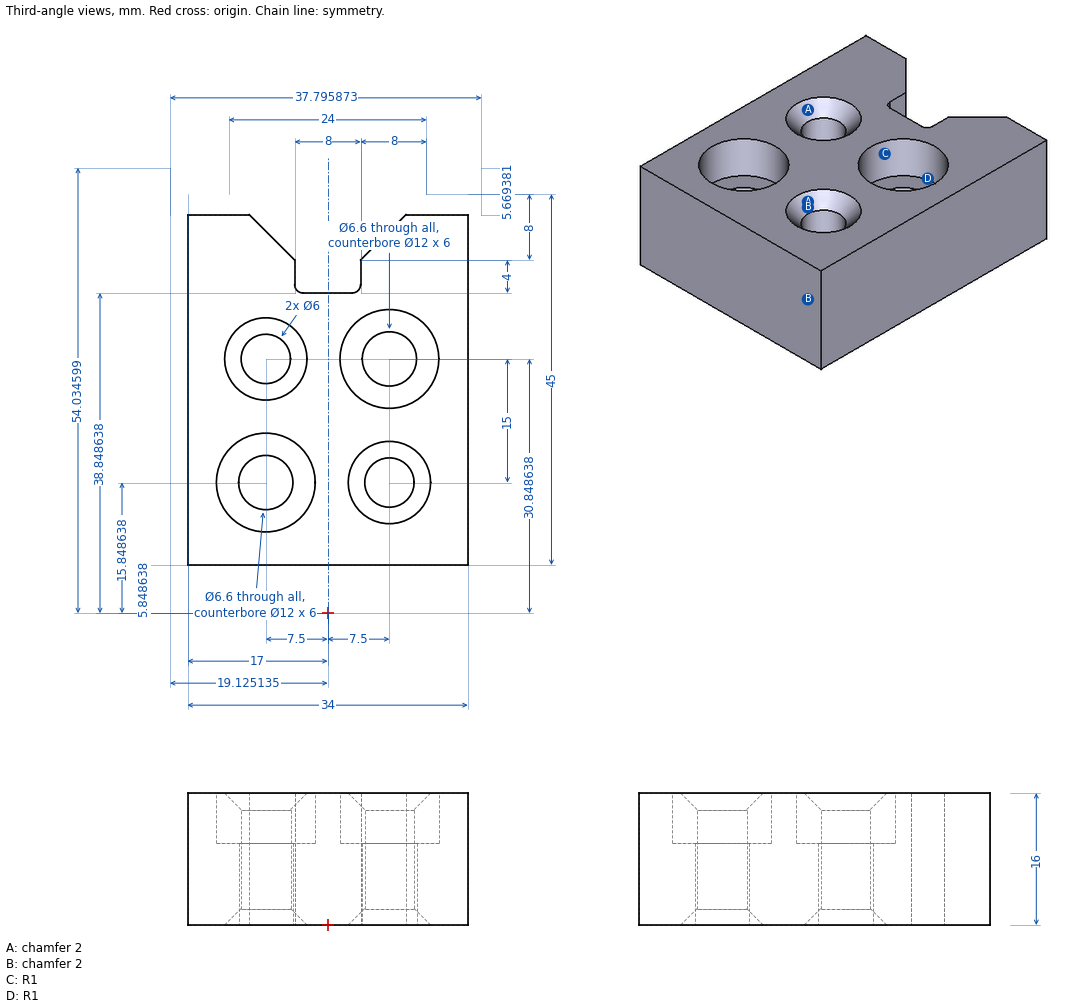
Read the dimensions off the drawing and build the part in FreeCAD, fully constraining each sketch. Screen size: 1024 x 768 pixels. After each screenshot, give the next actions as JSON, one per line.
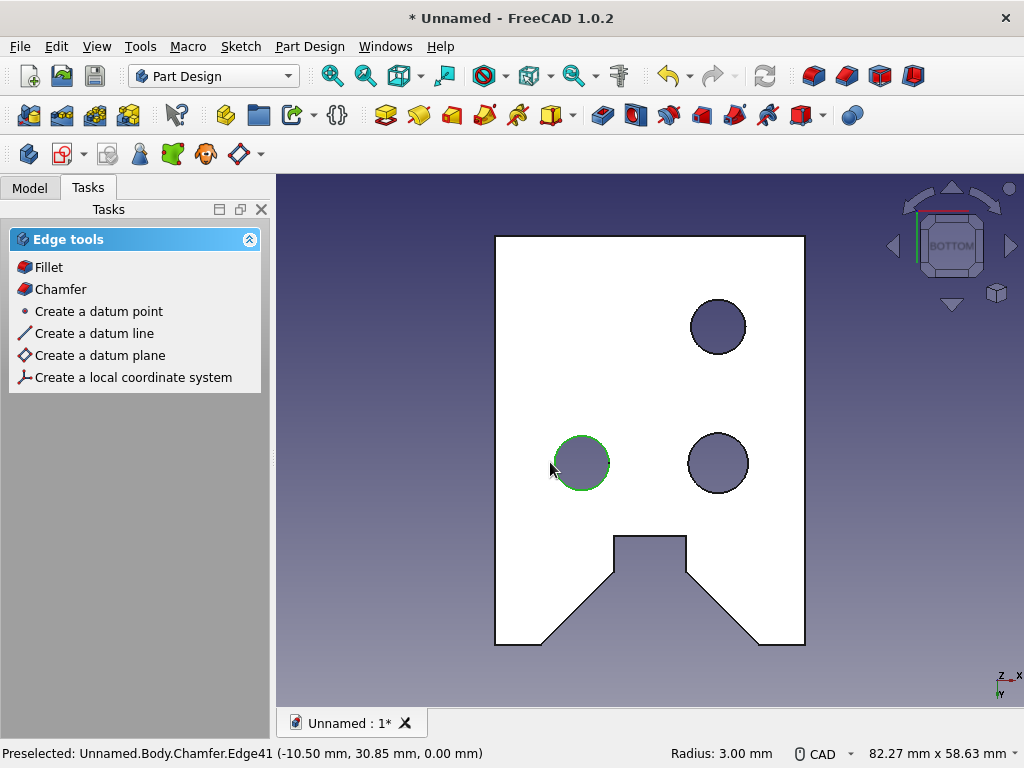
{"action": "left_click", "coordinate": [691, 326], "text": "ctrl"}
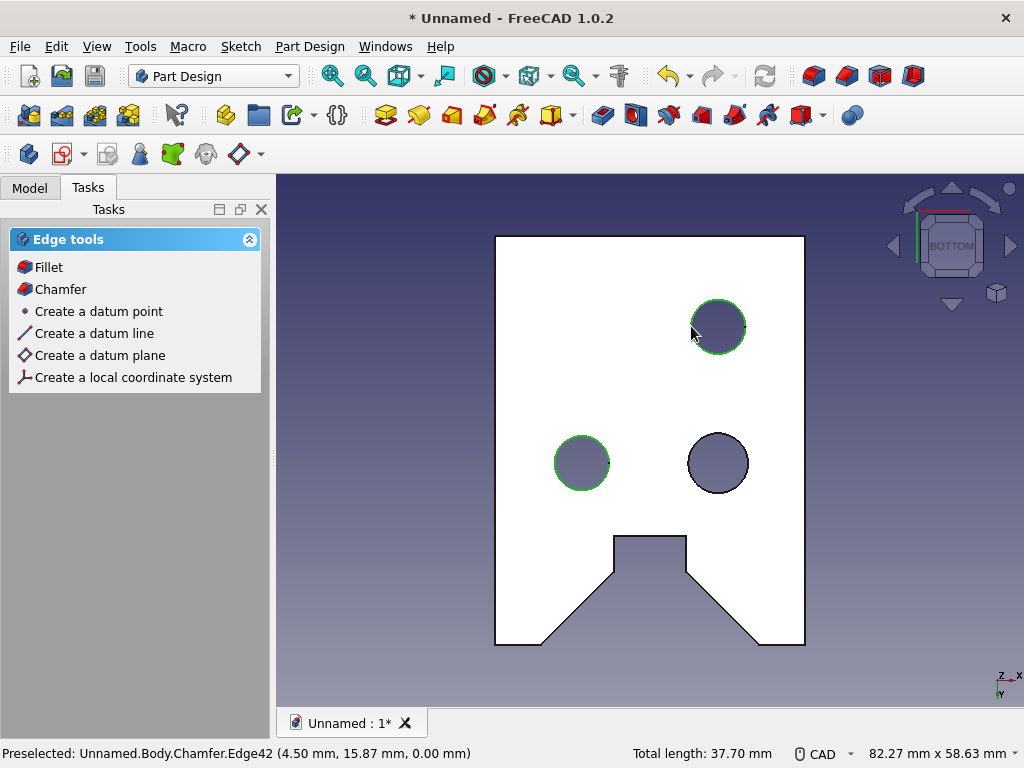
{"action": "left_click", "coordinate": [847, 76]}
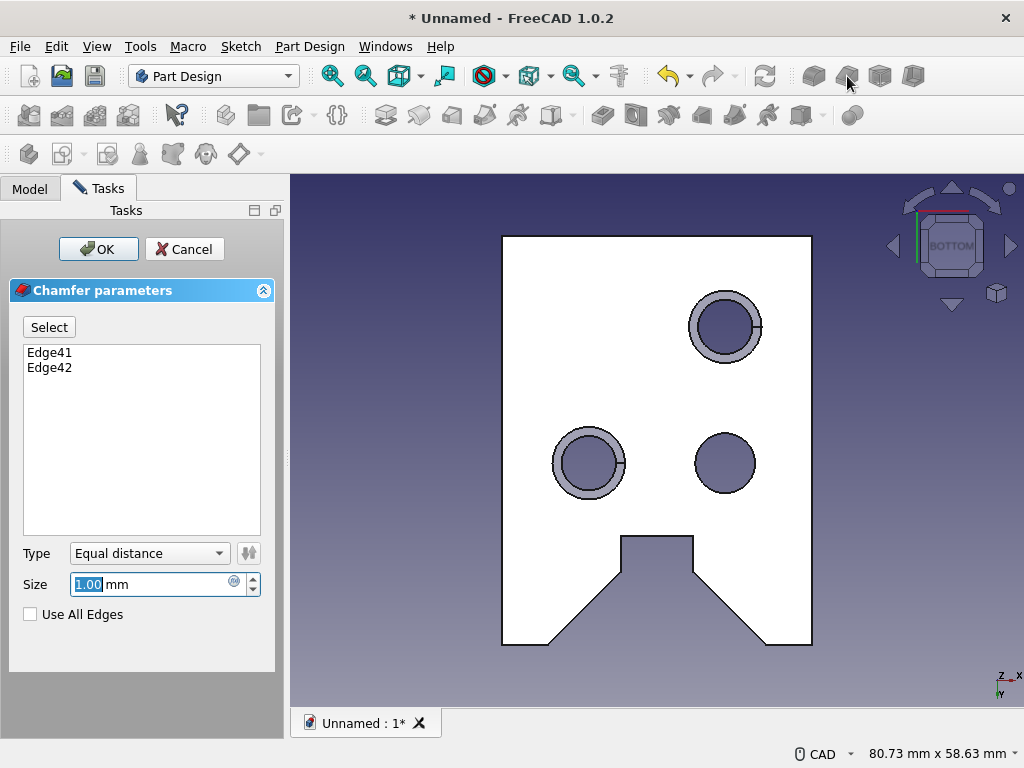
{"action": "type", "text": "2"}
{"action": "key", "text": "Tab"}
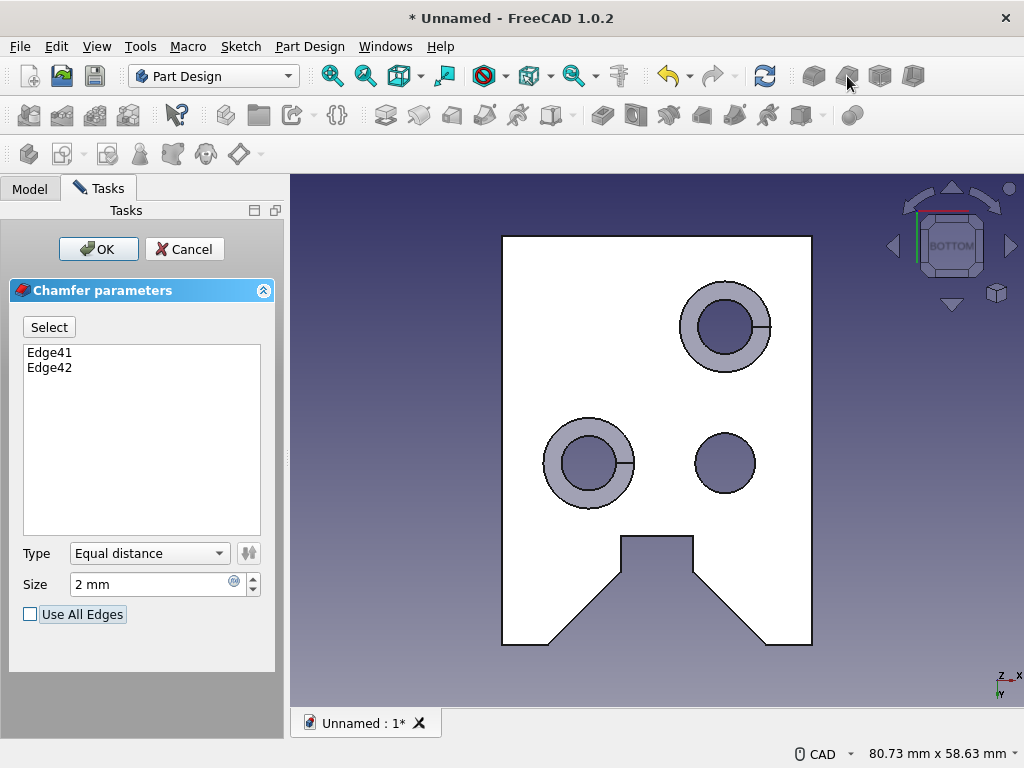
{"action": "left_click", "coordinate": [99, 249]}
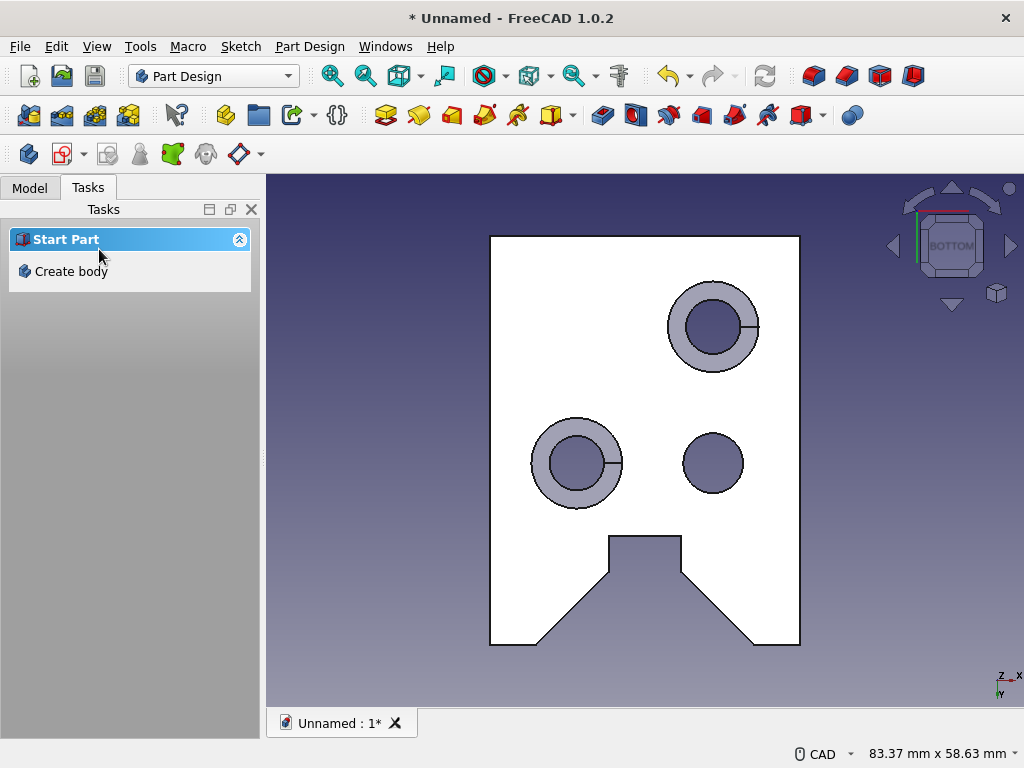
{"action": "key", "text": "0"}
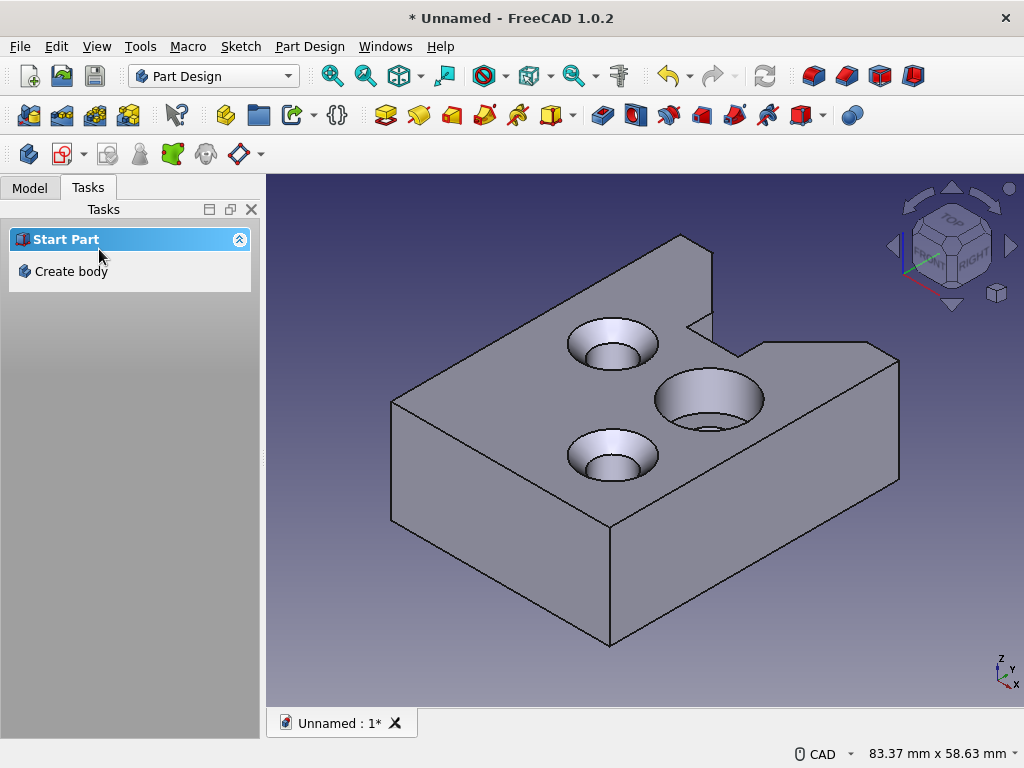
{"action": "left_click", "coordinate": [531, 410]}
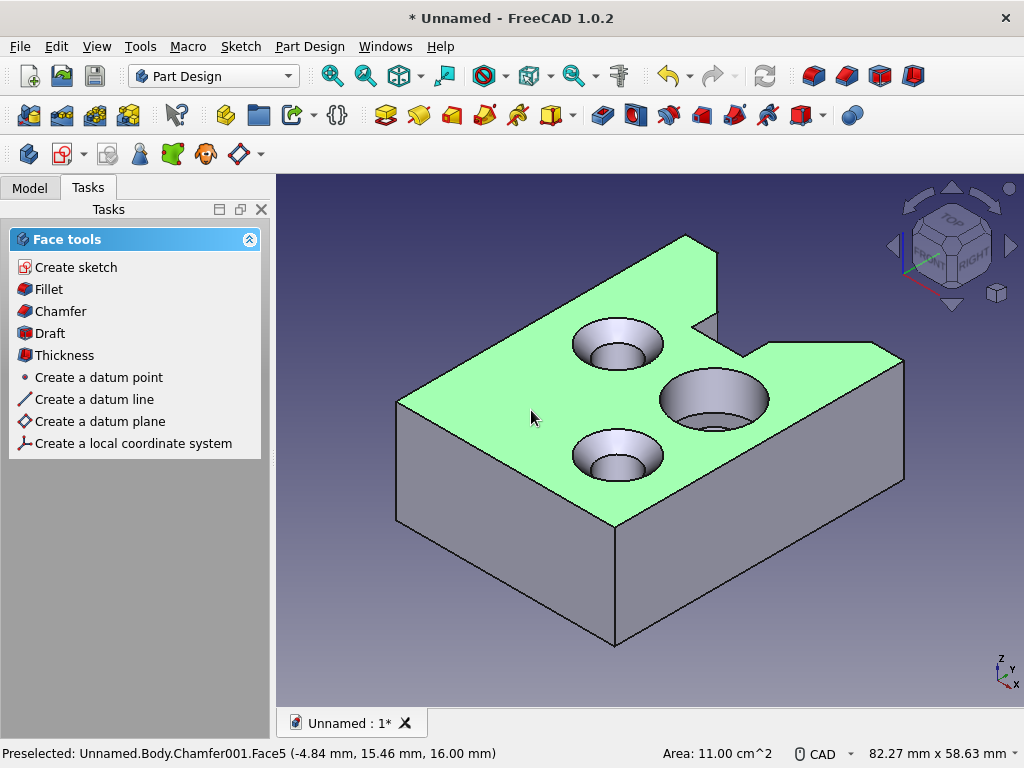
{"action": "left_click", "coordinate": [62, 154]}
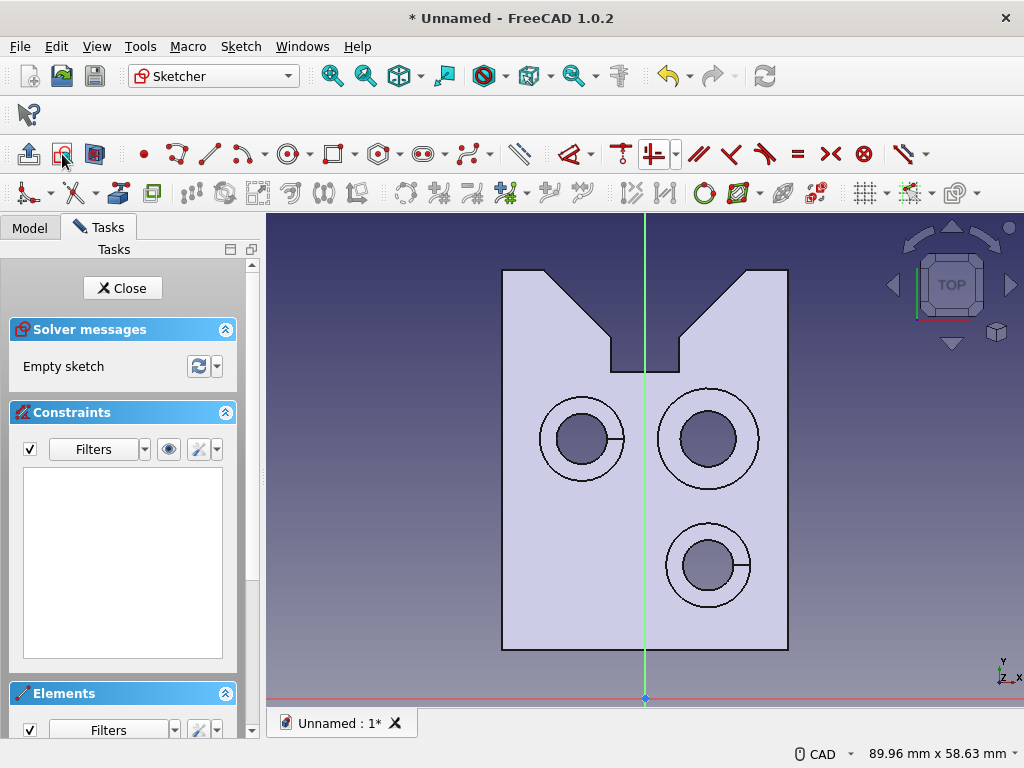
{"action": "scroll", "coordinate": [583, 586], "scroll_direction": "up", "scroll_amount": 9}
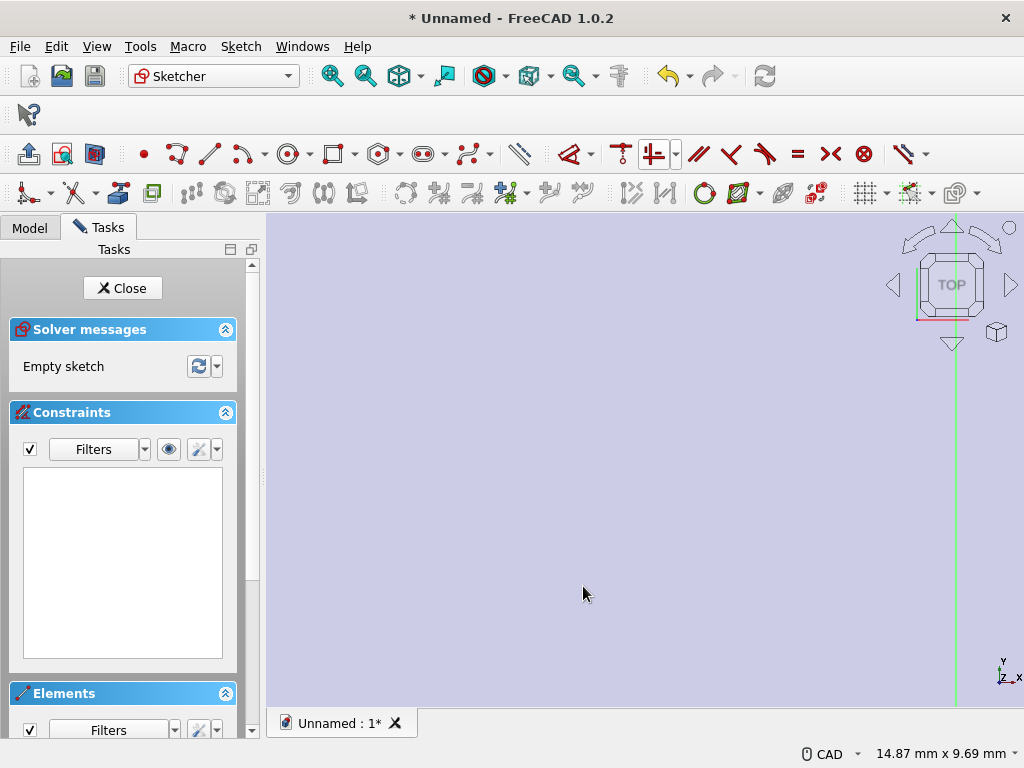
{"action": "left_click", "coordinate": [288, 154]}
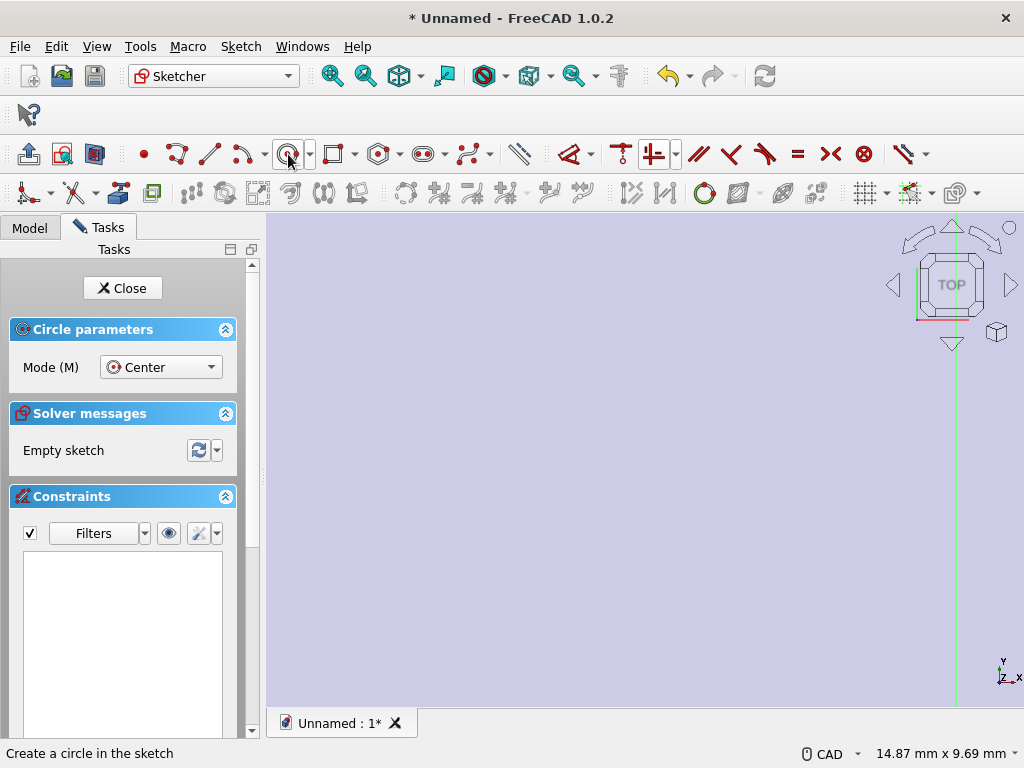
{"action": "left_click", "coordinate": [574, 457]}
{"action": "mouse_move", "coordinate": [693, 338]}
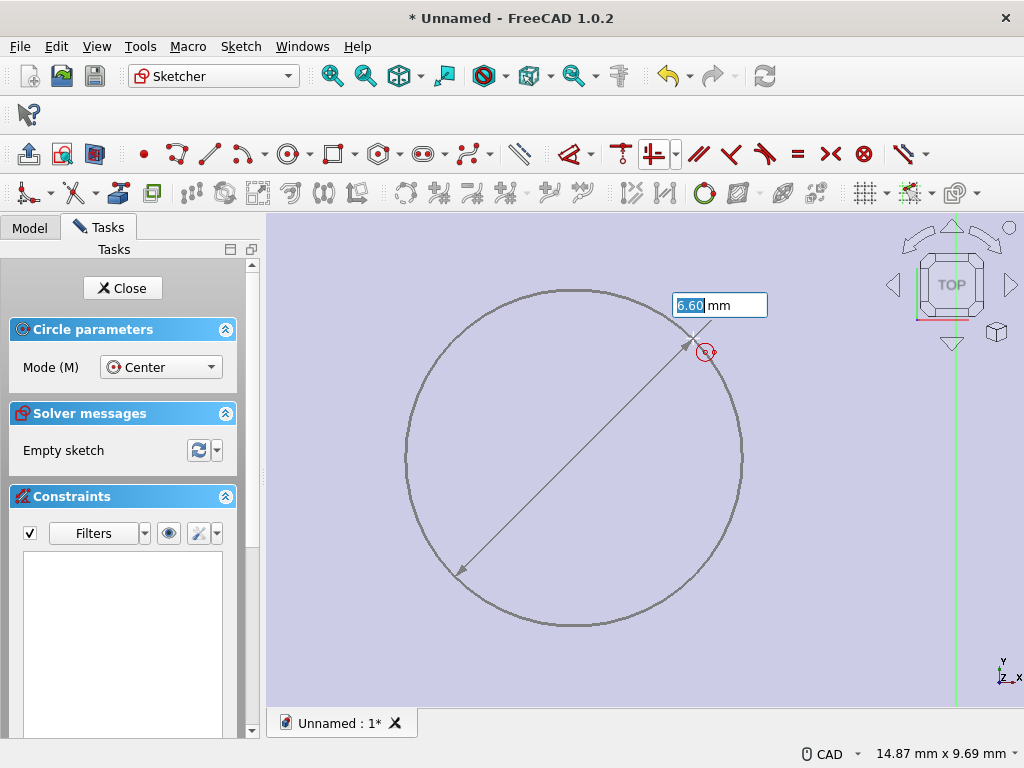
{"action": "type", "text": "6.6"}
{"action": "key", "text": "Return"}
{"action": "key", "text": "Escape"}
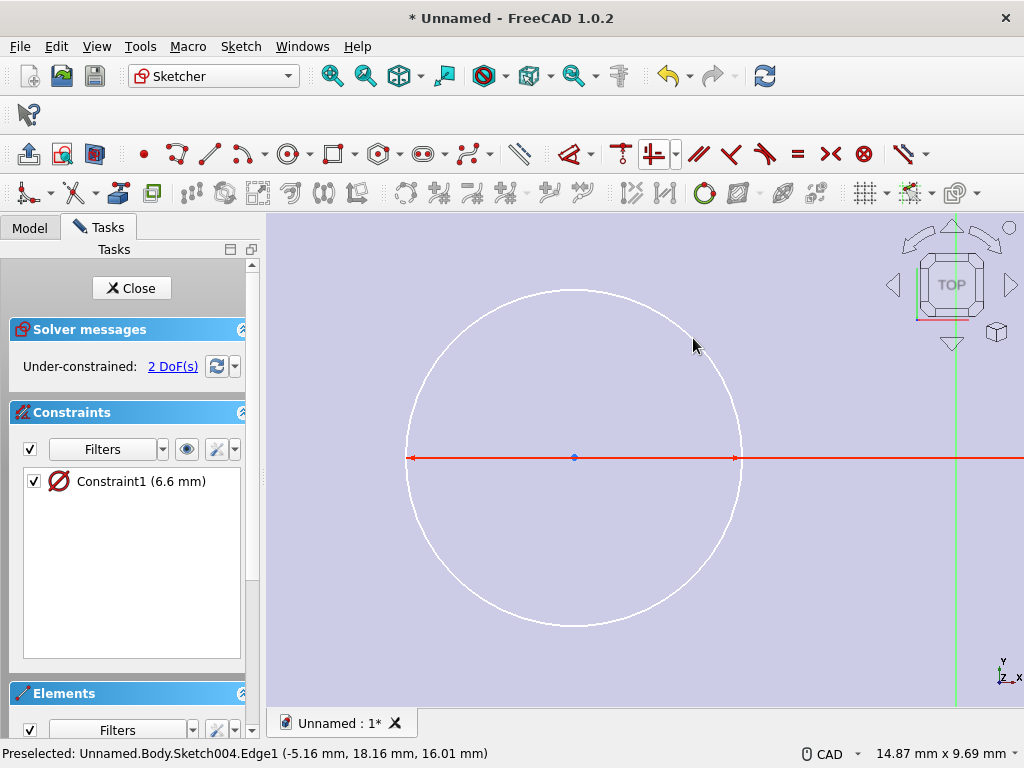
{"action": "left_click", "coordinate": [568, 154]}